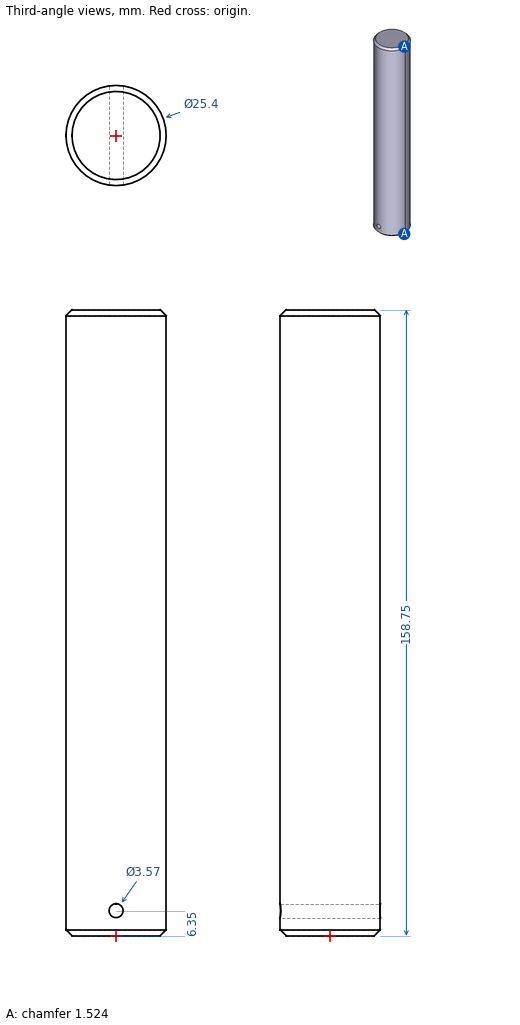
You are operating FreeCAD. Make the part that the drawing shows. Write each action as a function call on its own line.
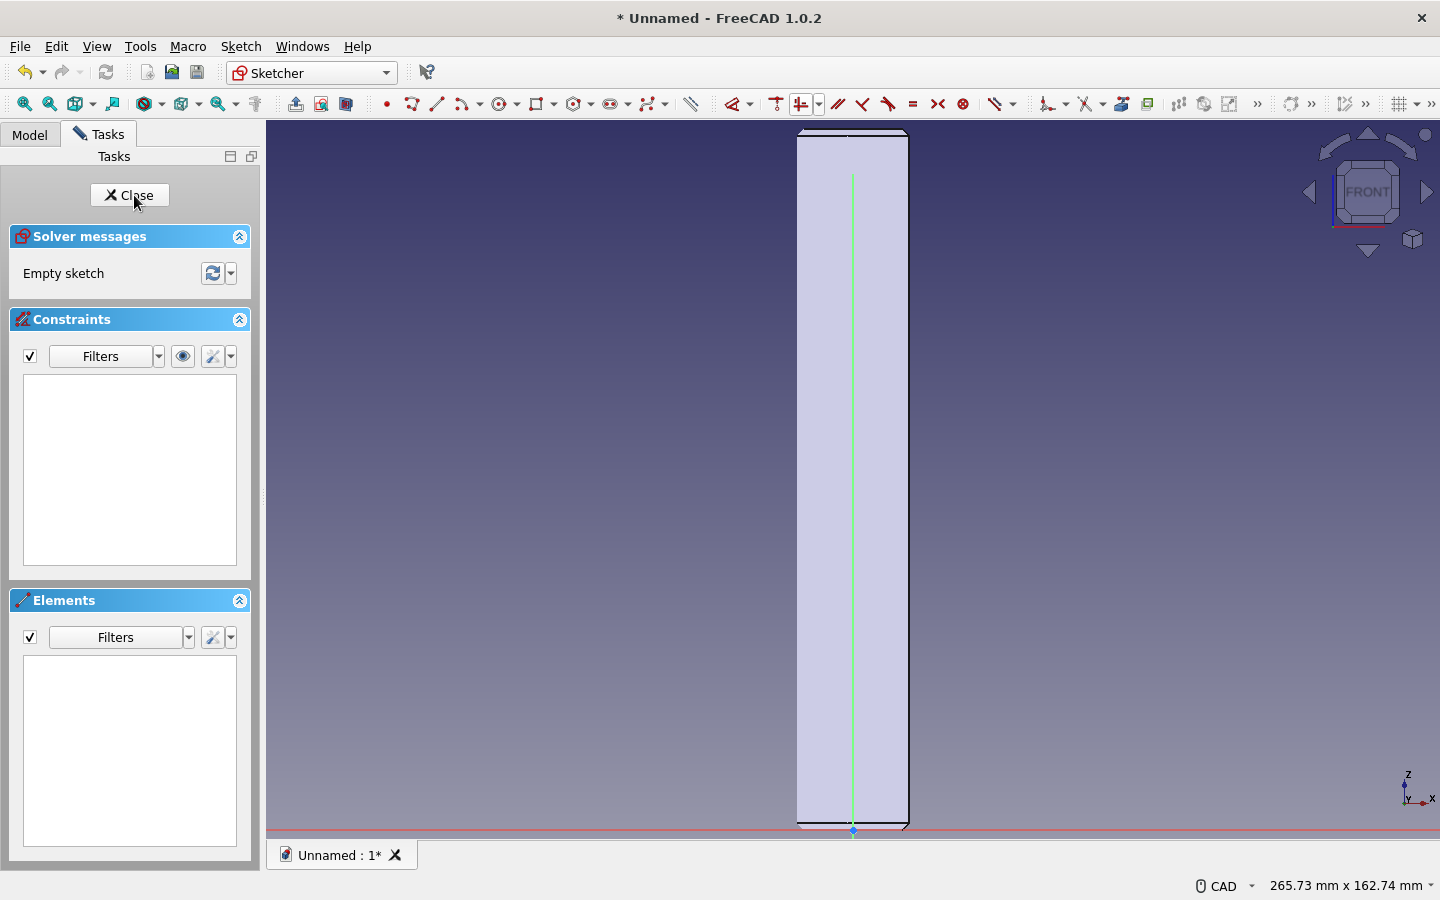
scroll(784, 480, down, 5)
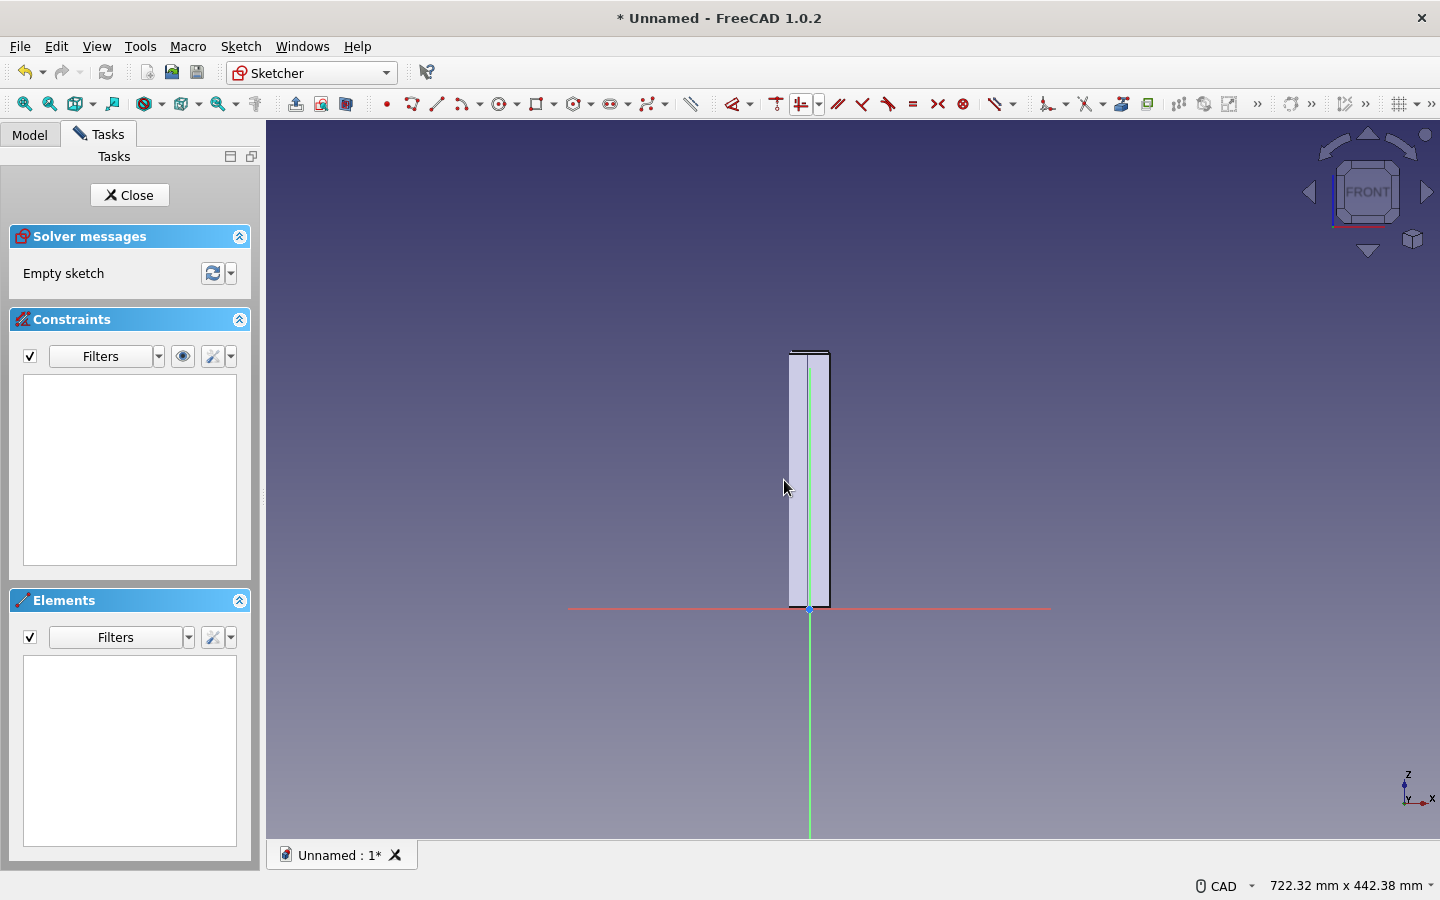
scroll(811, 609, up, 15)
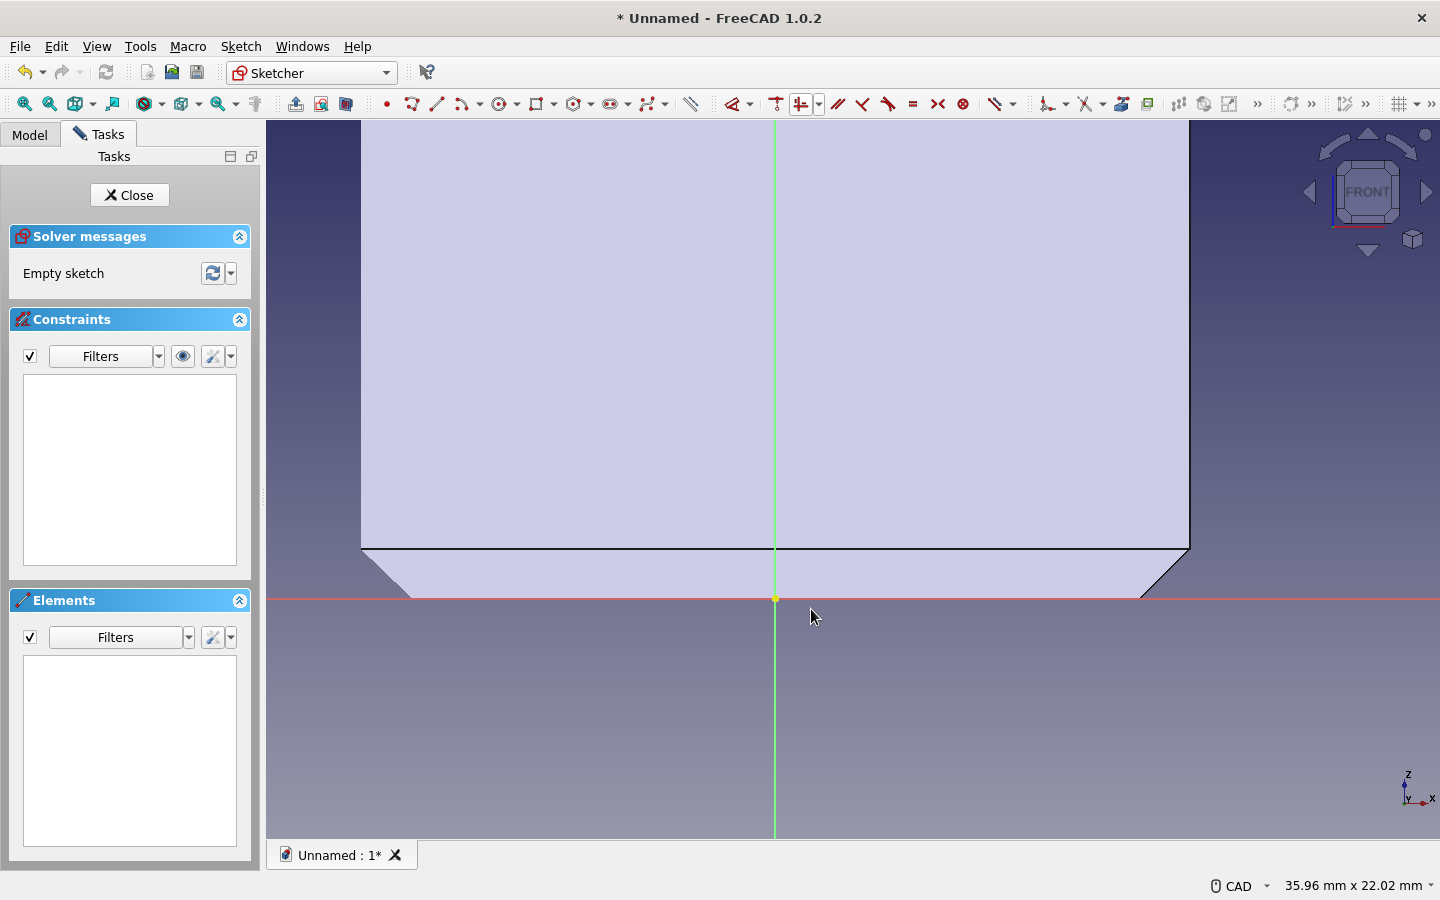
scroll(764, 450, up, 3)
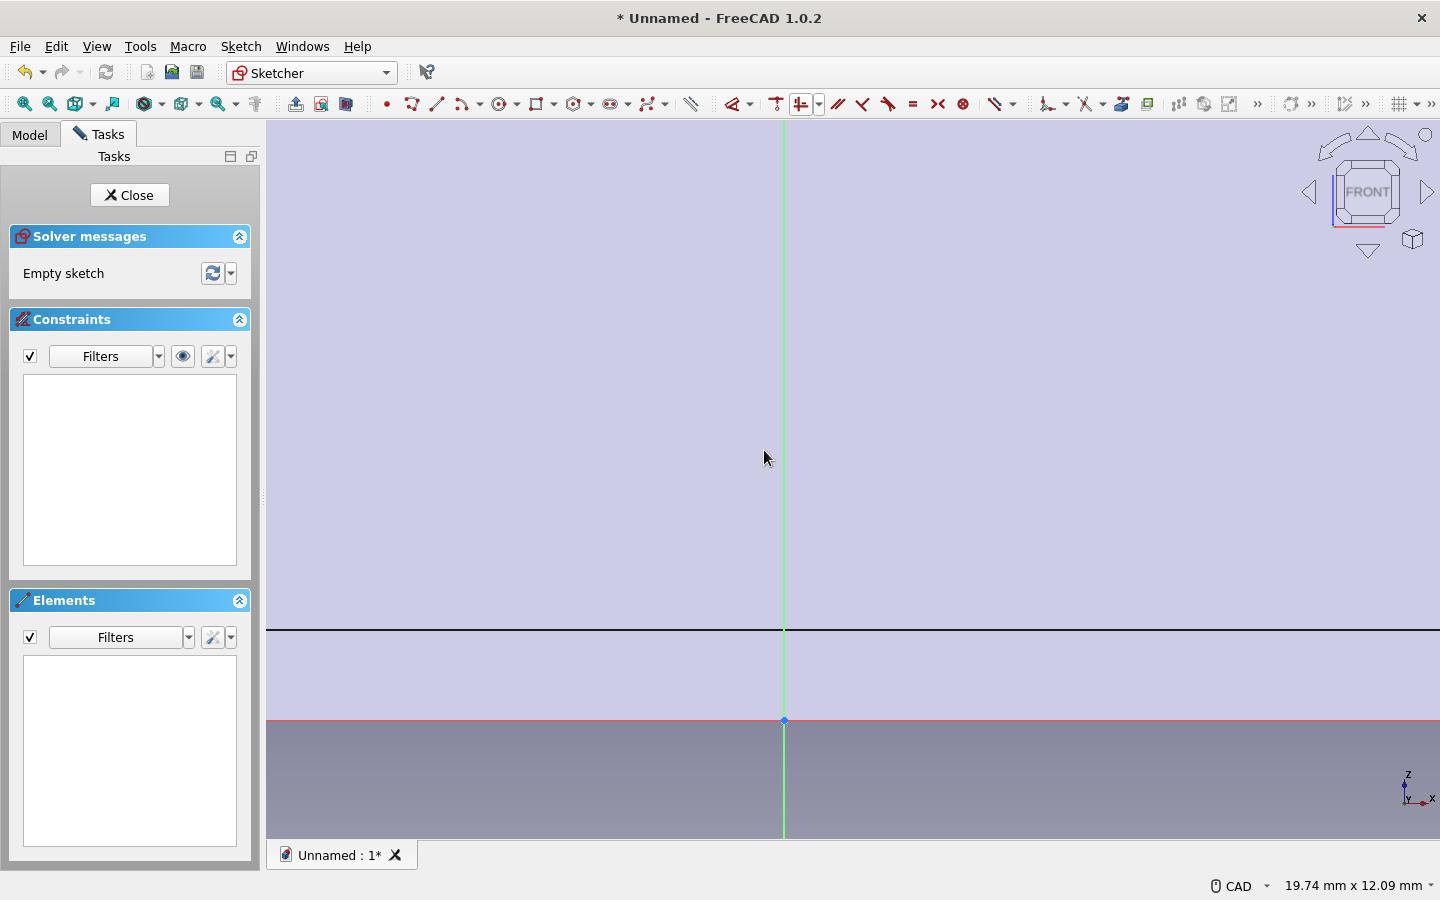
key(g)
key(c)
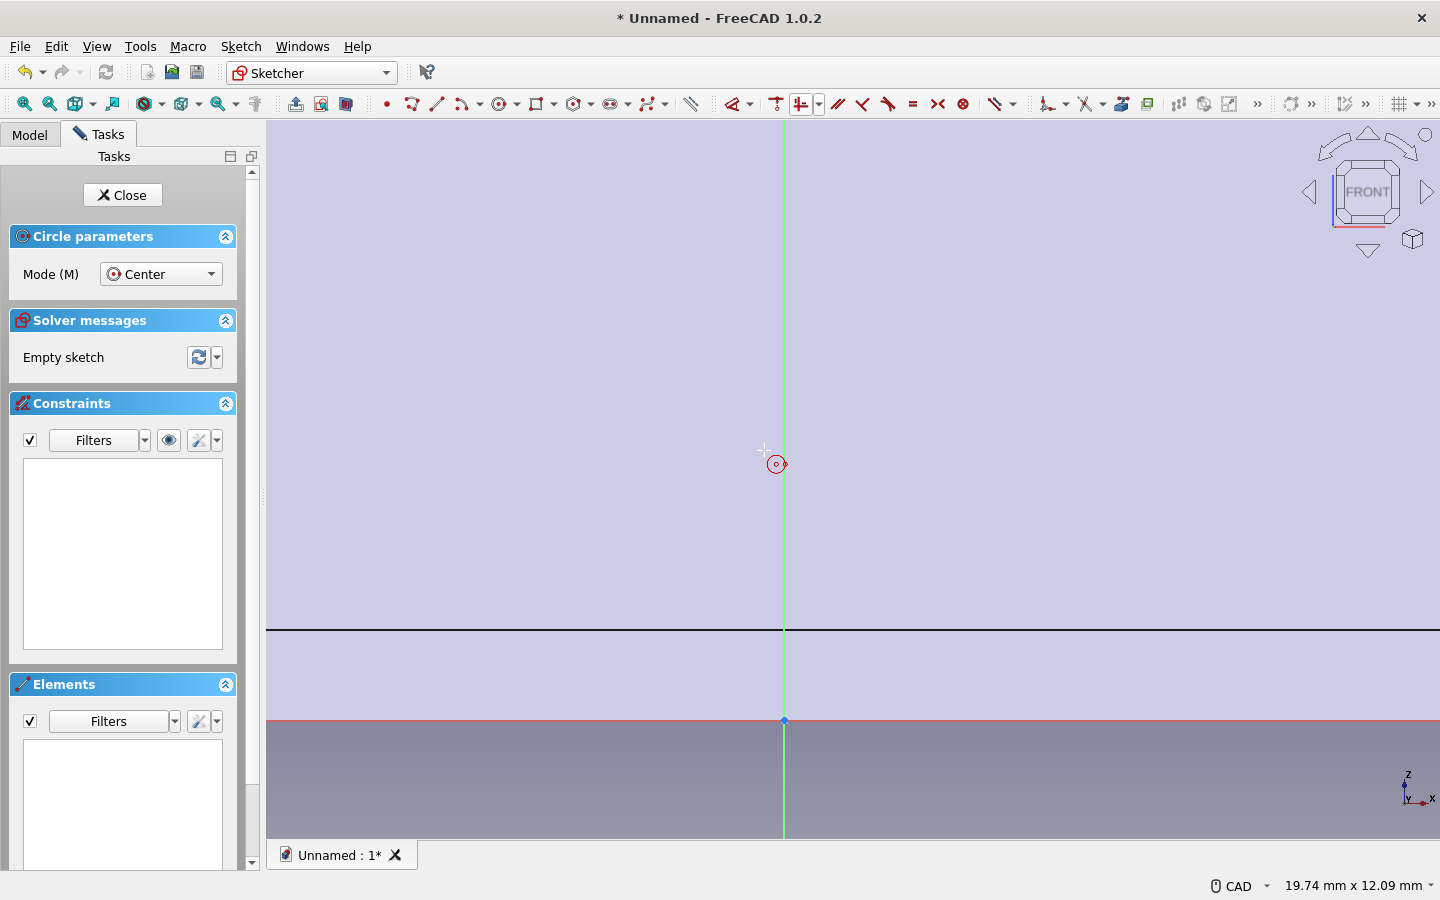
click(784, 343)
click(859, 268)
key(Escape)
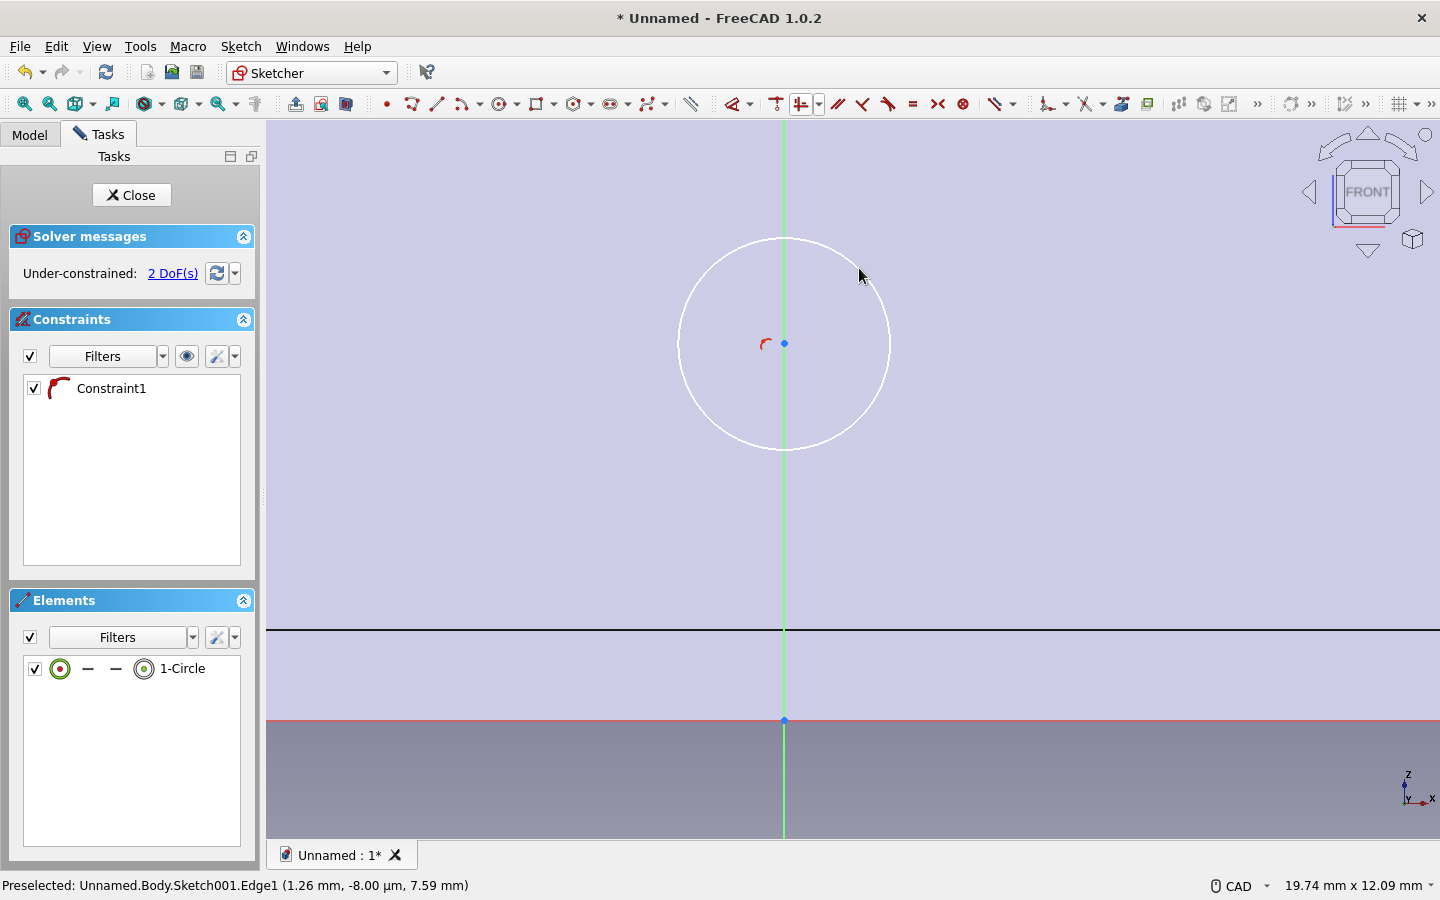
click(859, 269)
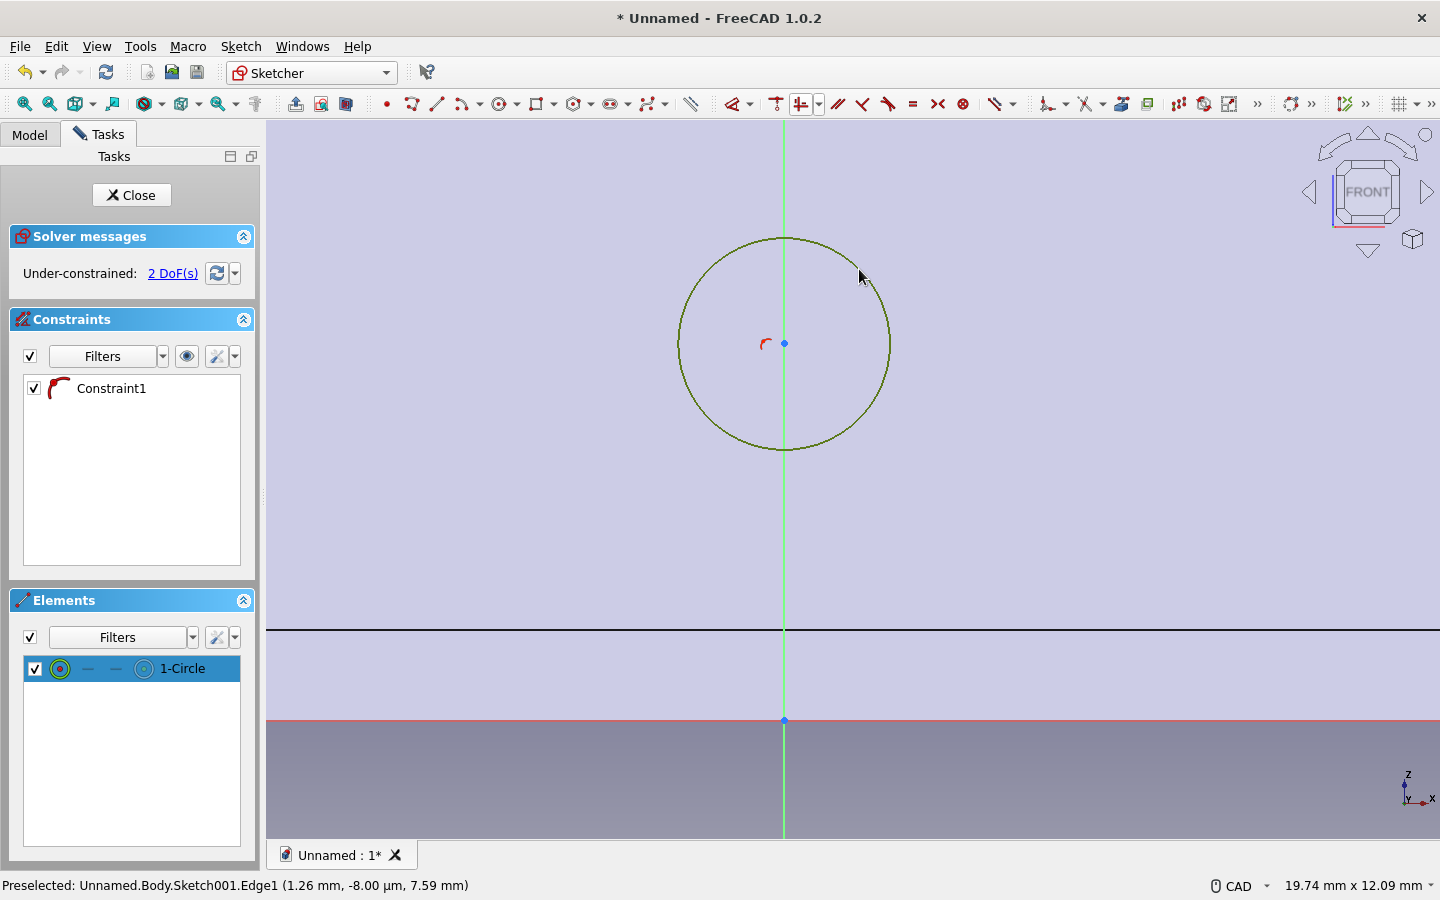
click(750, 104)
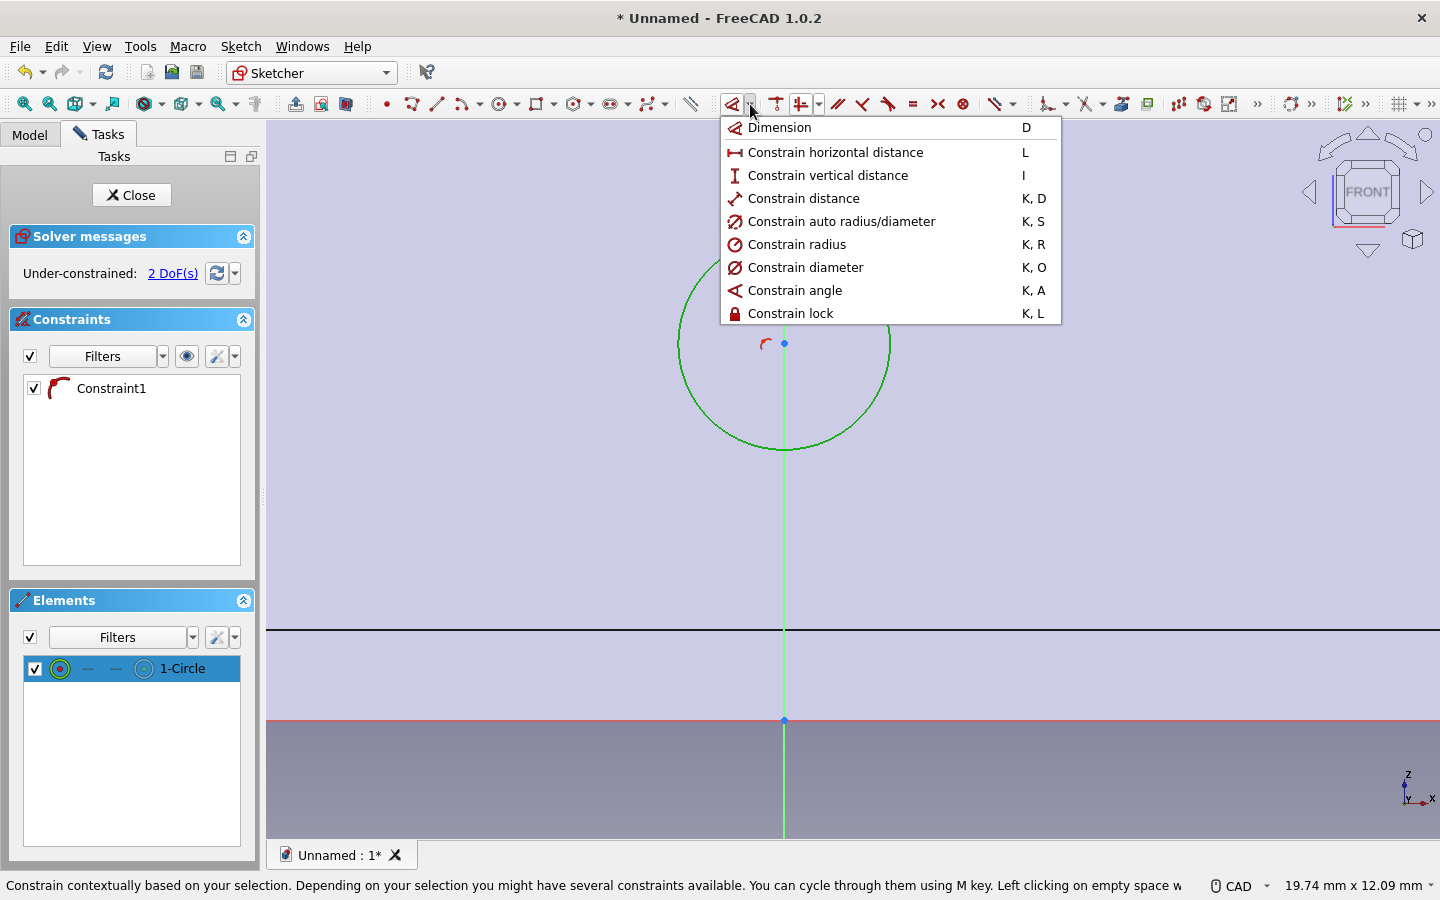
click(891, 268)